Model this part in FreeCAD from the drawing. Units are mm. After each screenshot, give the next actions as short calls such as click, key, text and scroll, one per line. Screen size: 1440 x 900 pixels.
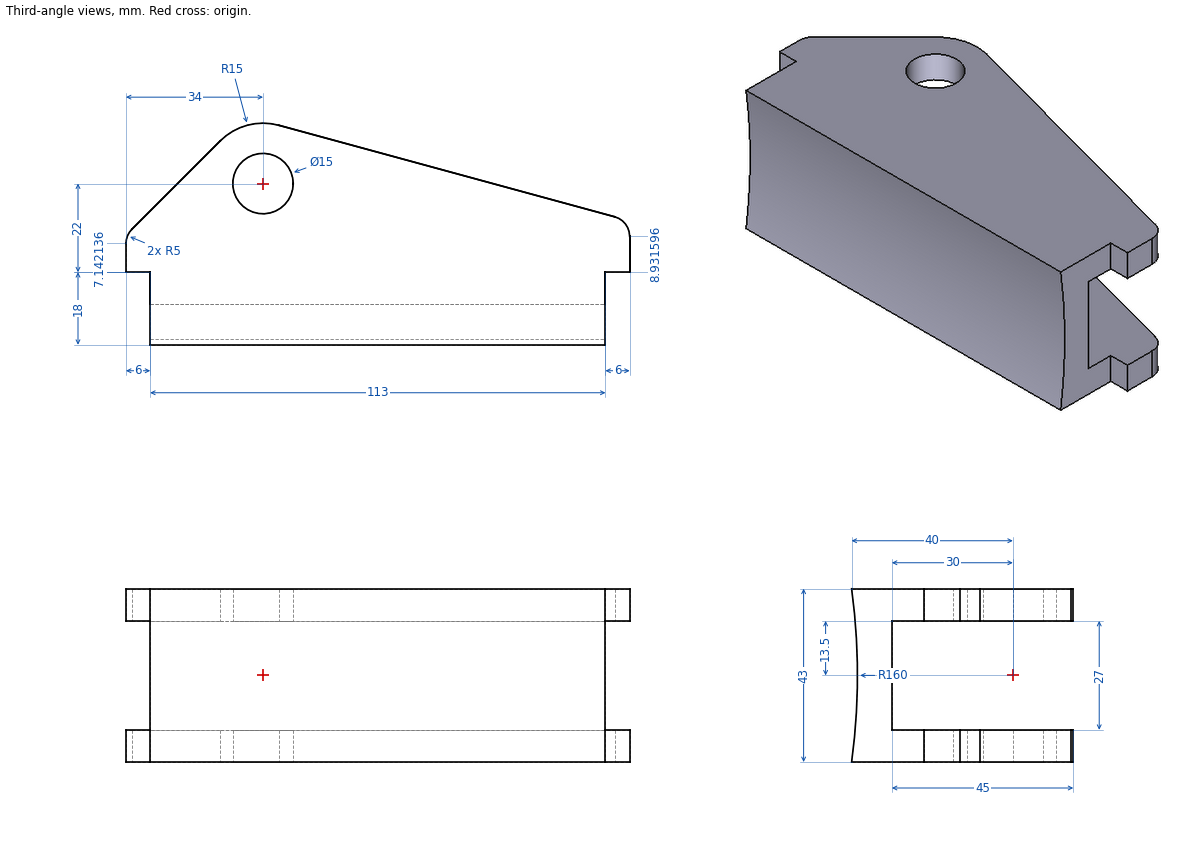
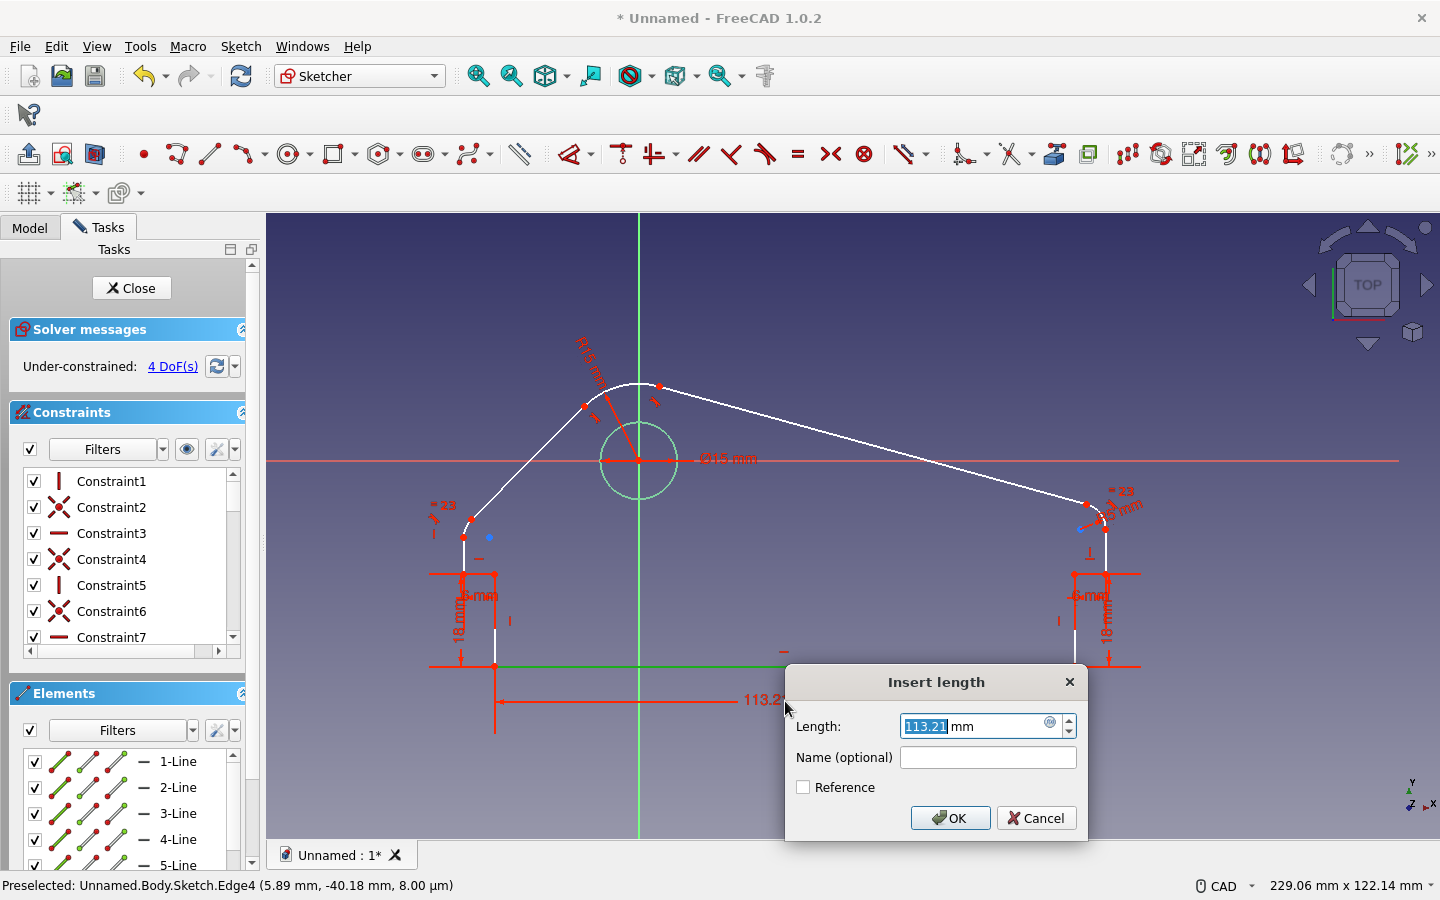
text(113)
key(Return)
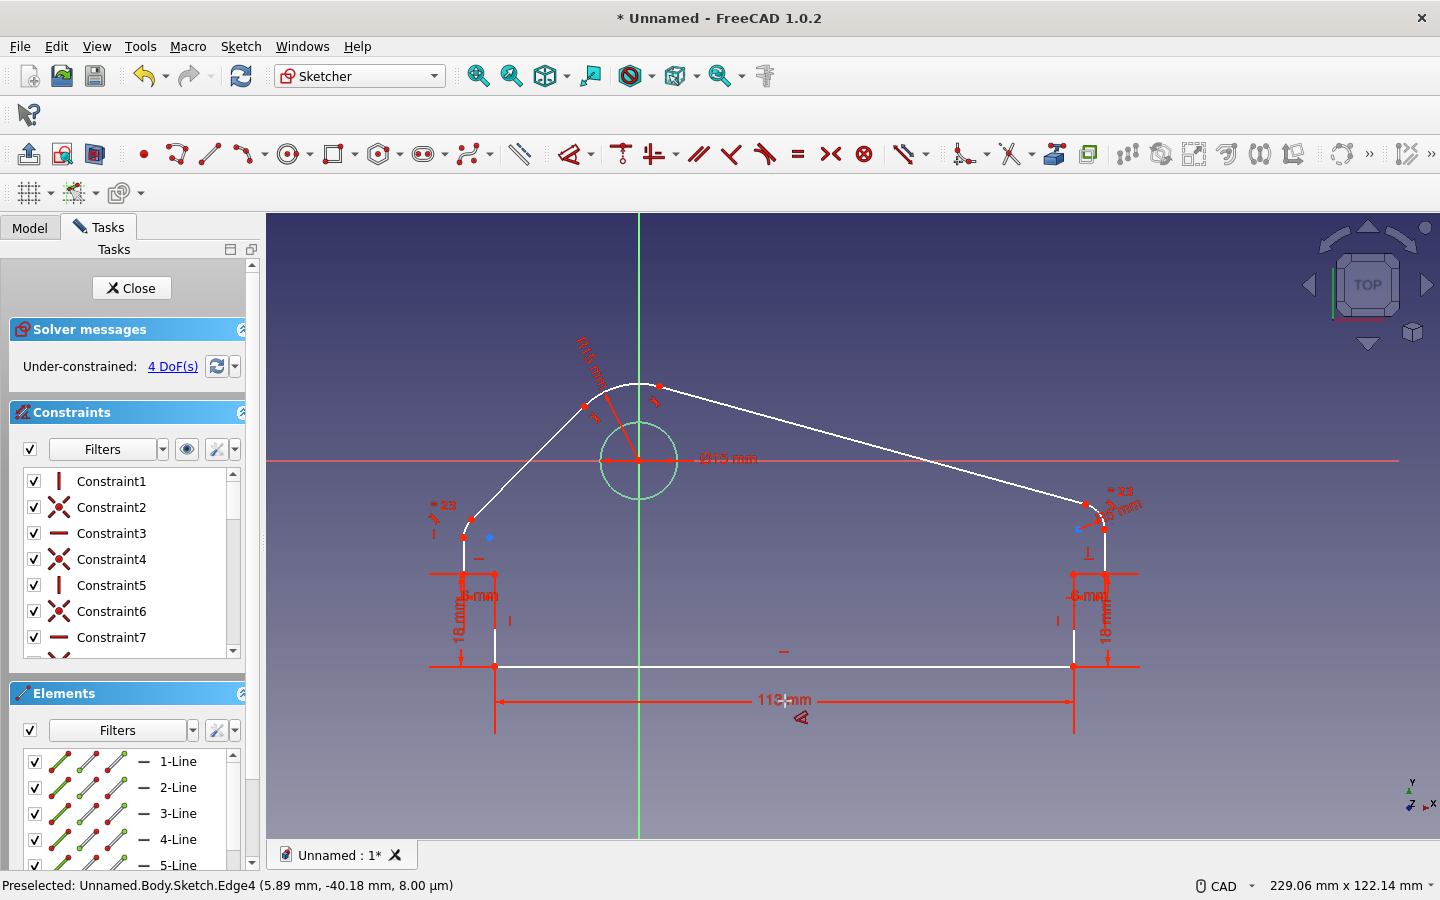
click(464, 538)
click(511, 427)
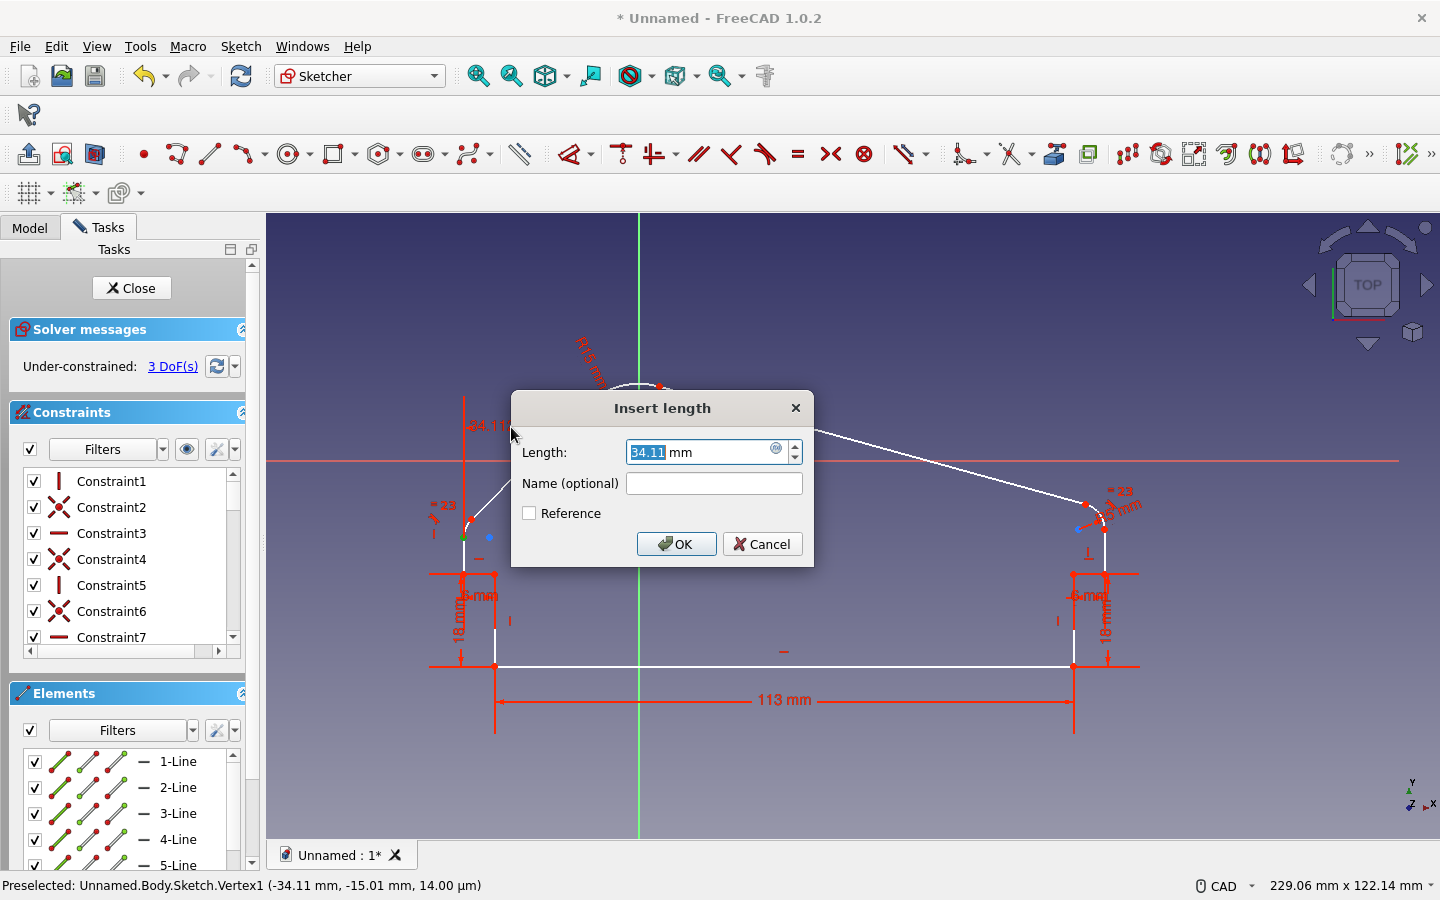
text(34)
key(Return)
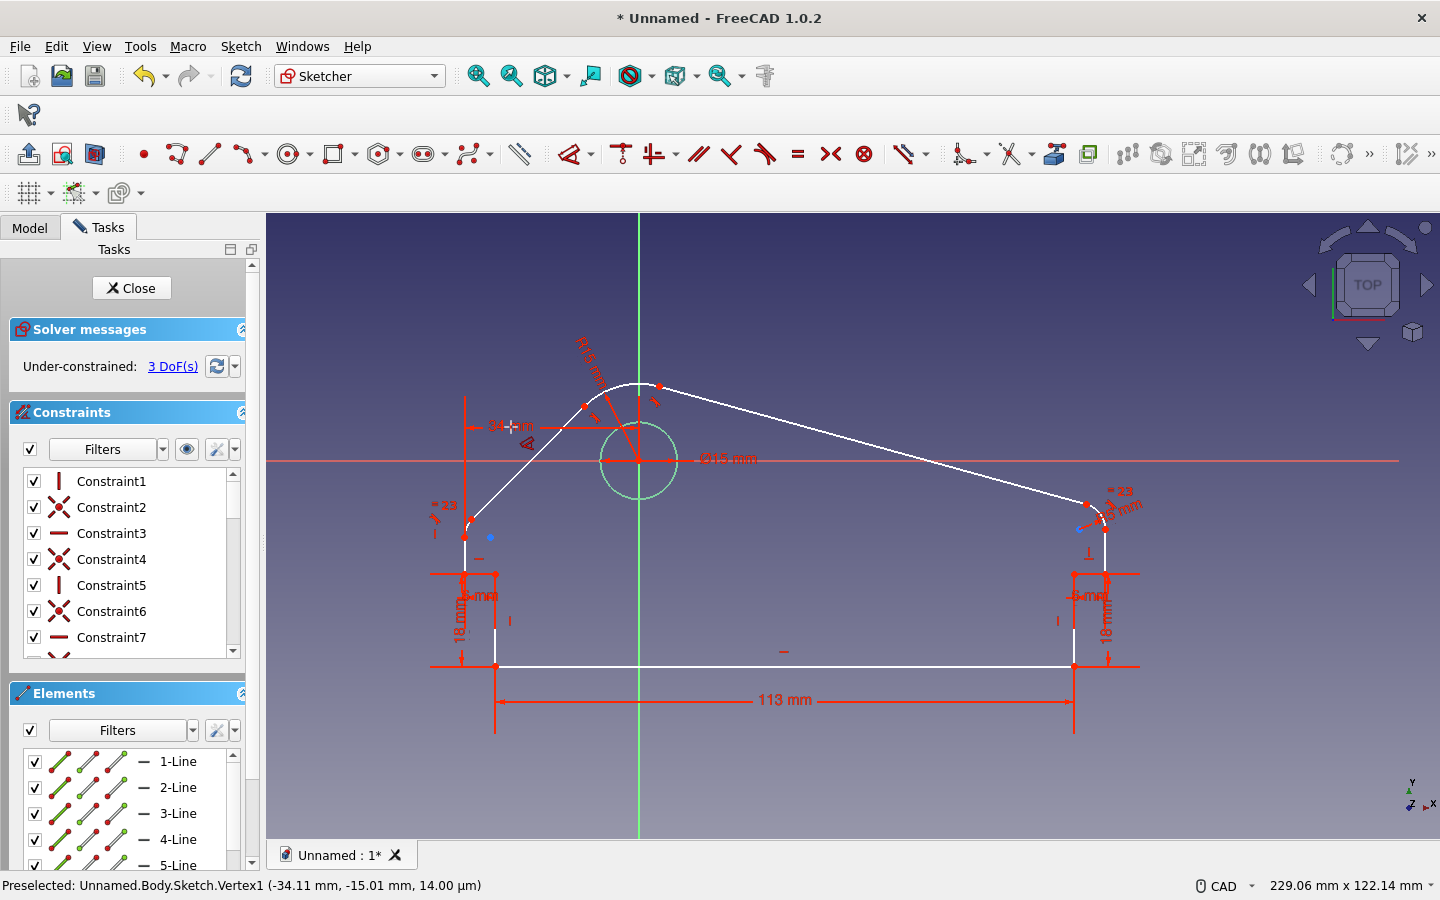
click(465, 574)
click(431, 518)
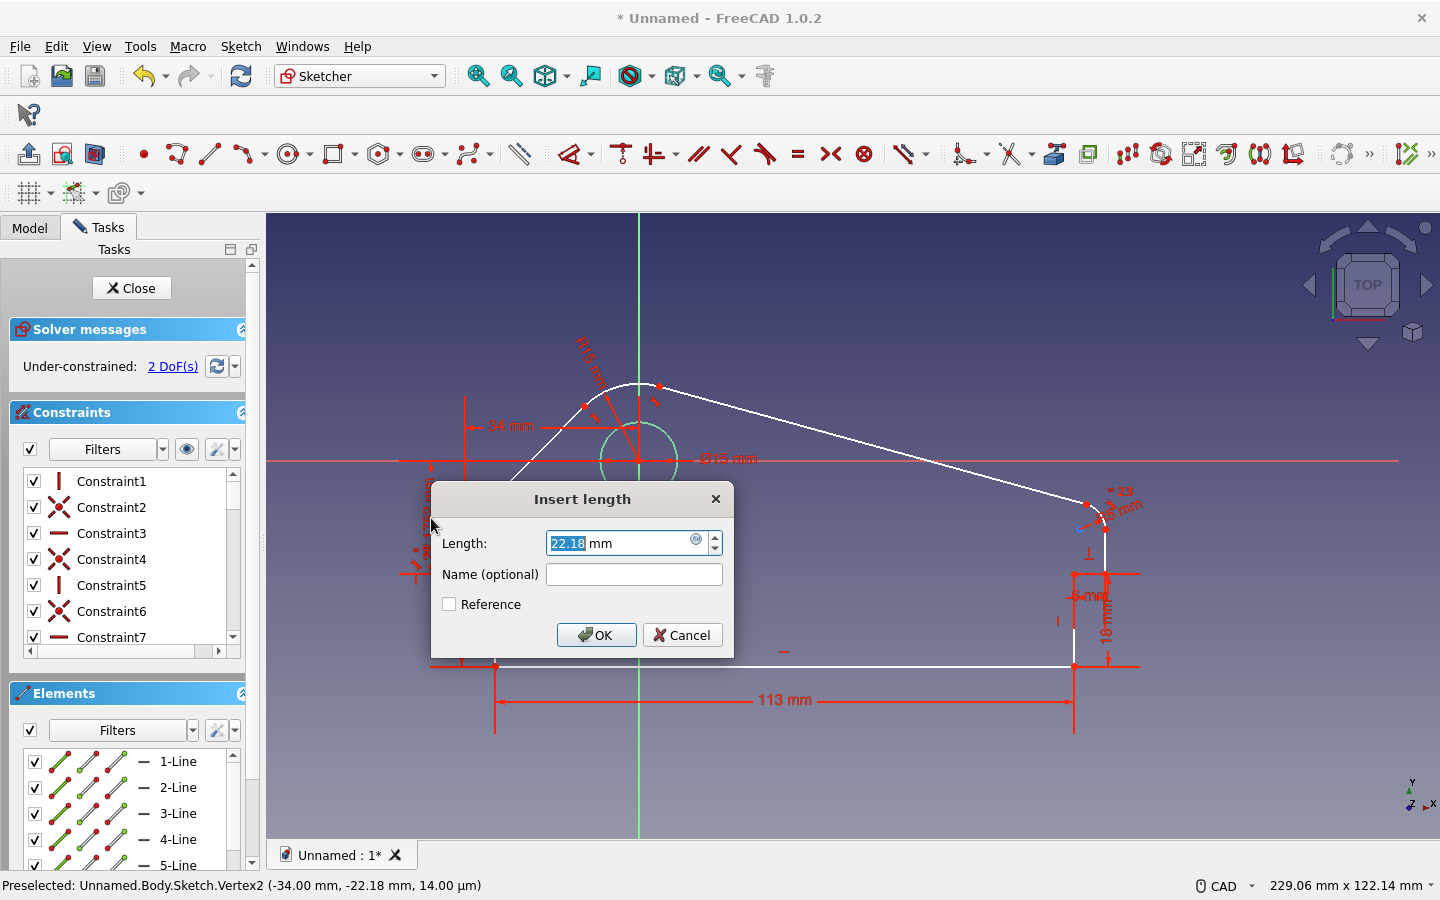
text(22)
key(Return)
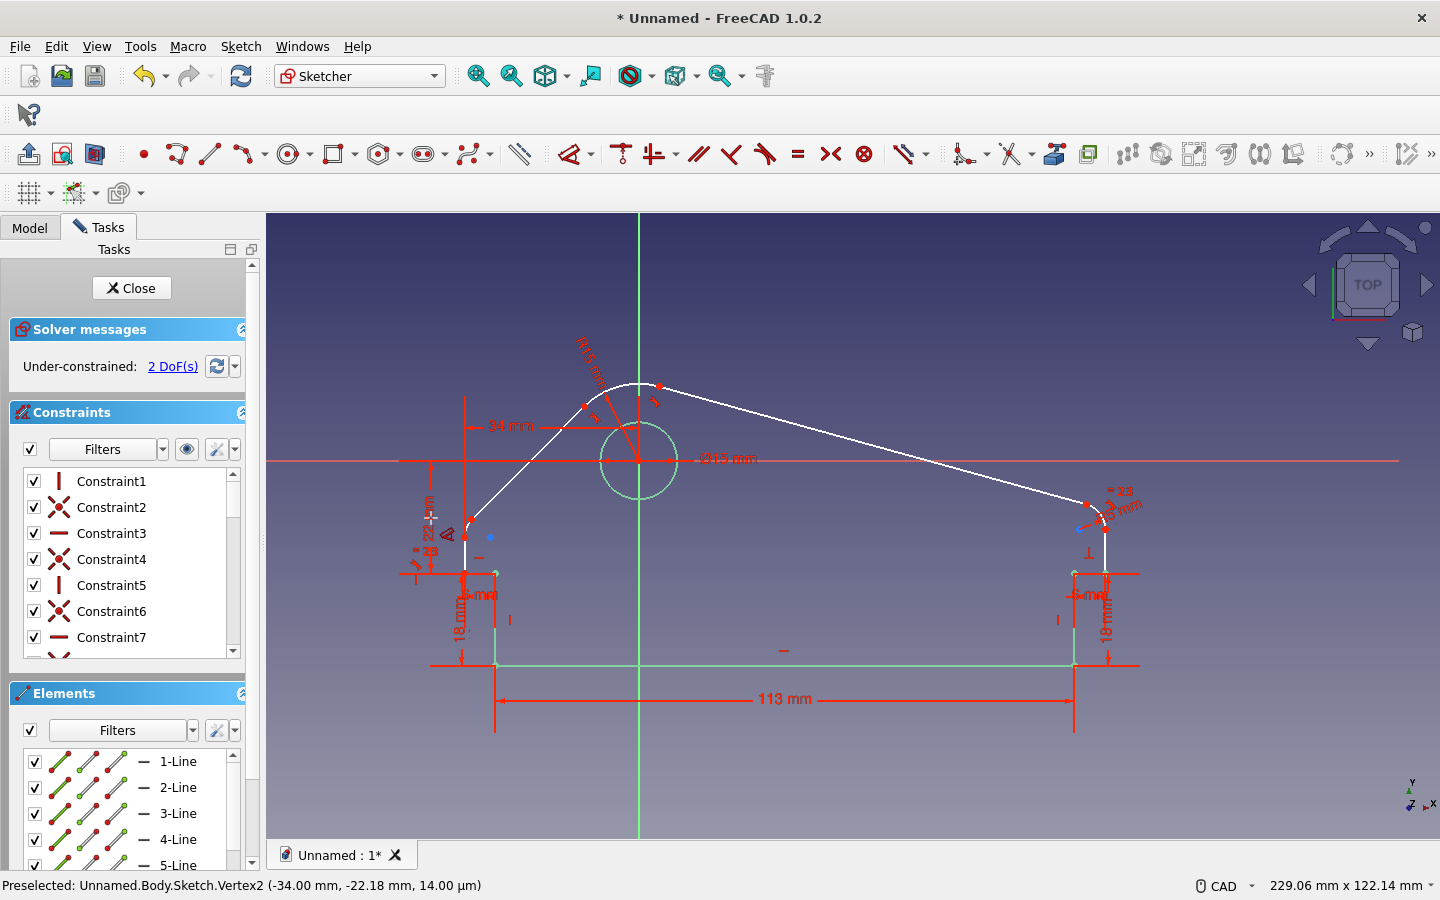
scroll(465, 548, up, 2)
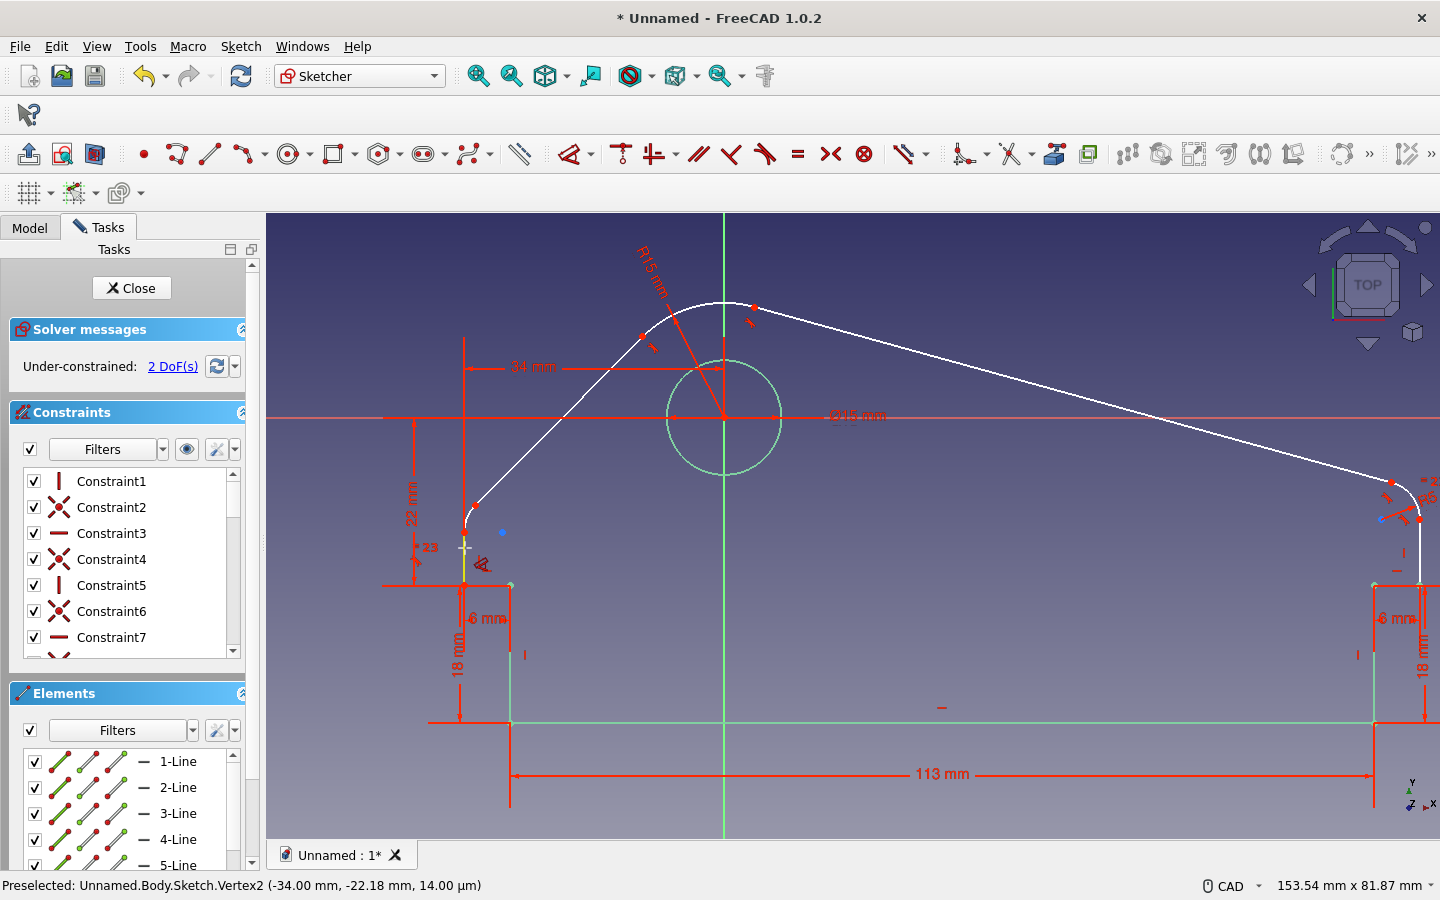
click(464, 548)
click(430, 559)